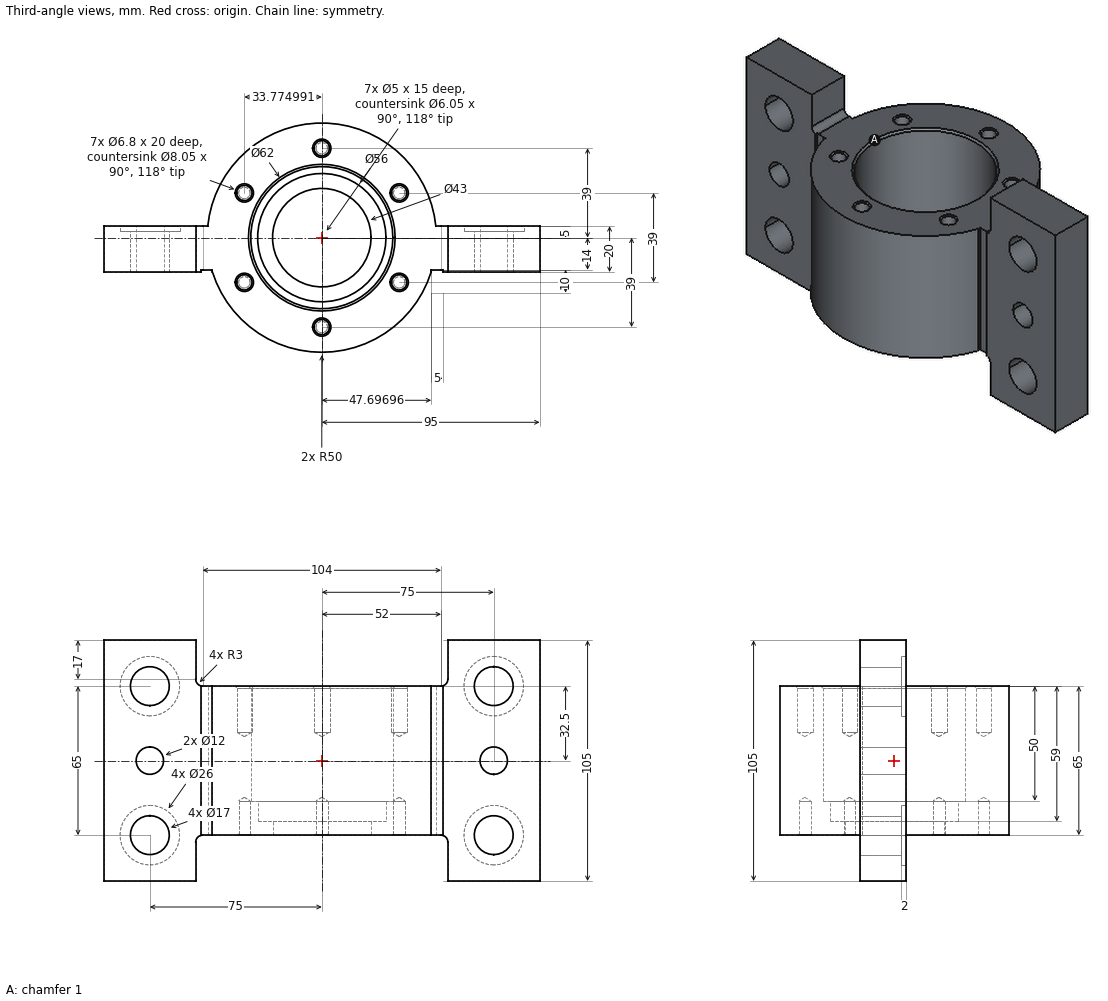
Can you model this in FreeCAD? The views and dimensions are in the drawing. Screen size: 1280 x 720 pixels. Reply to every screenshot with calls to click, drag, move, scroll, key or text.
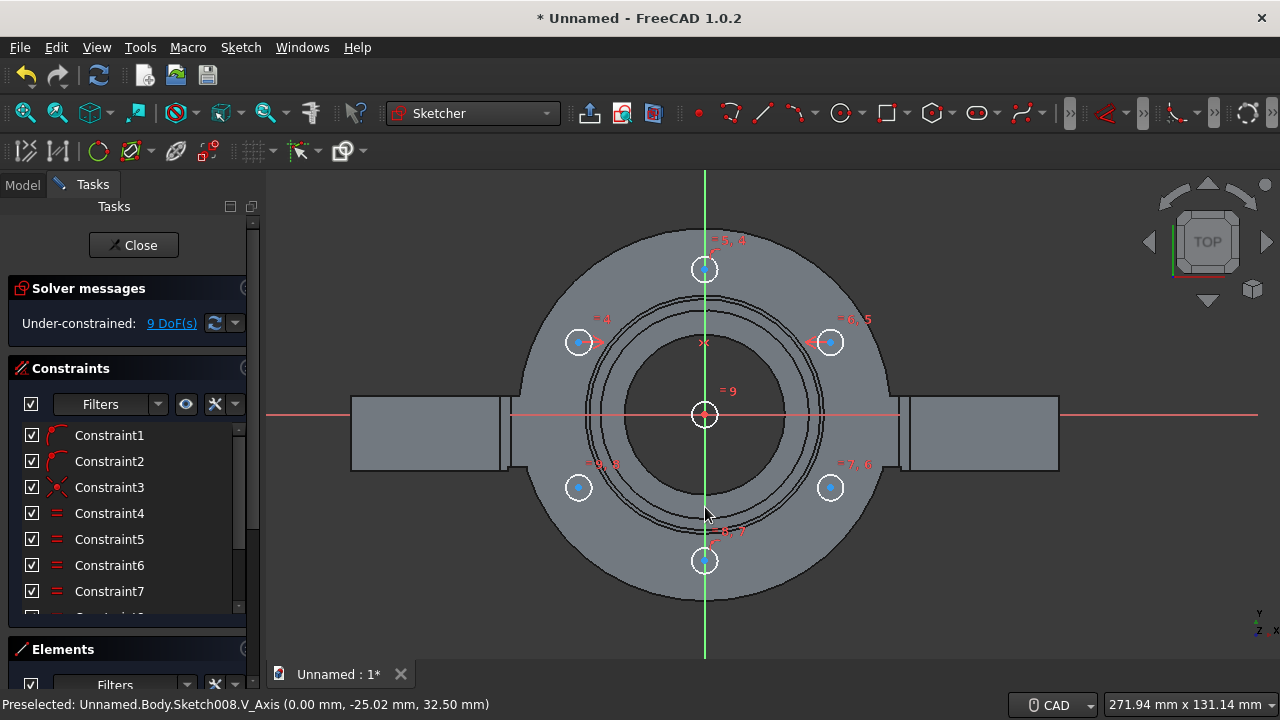
click(831, 342)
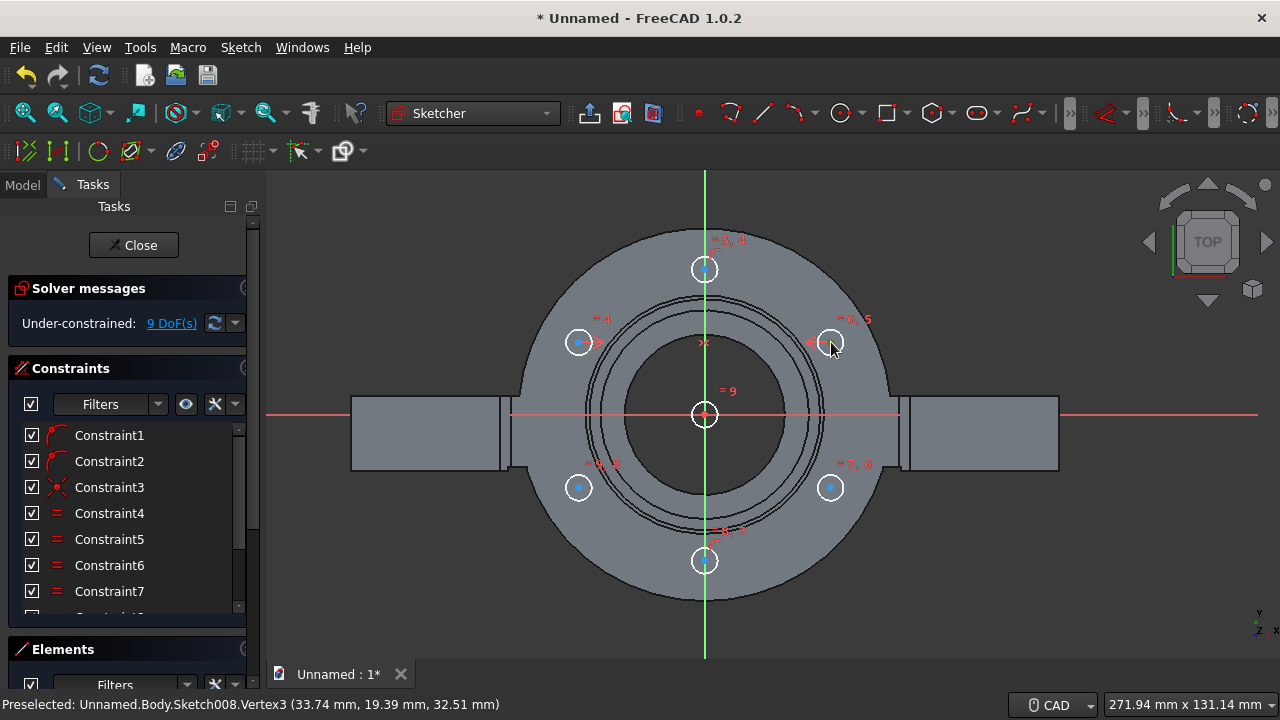
click(831, 488)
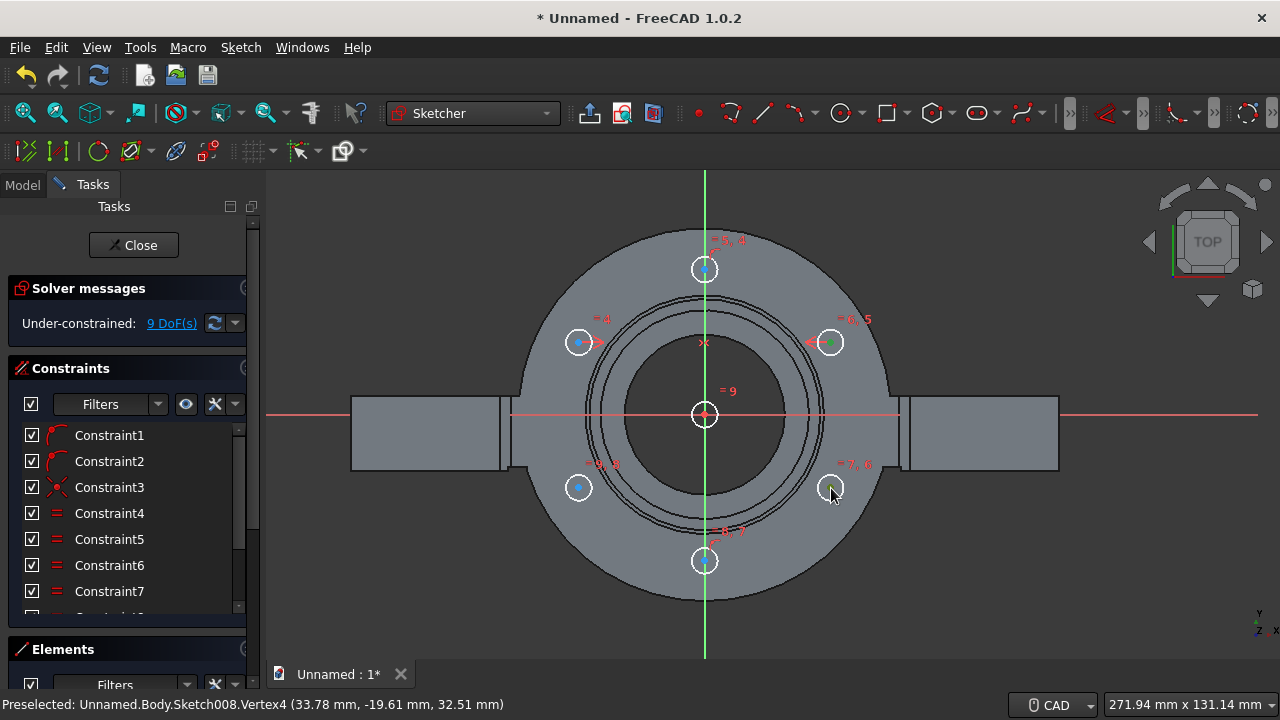
click(353, 415)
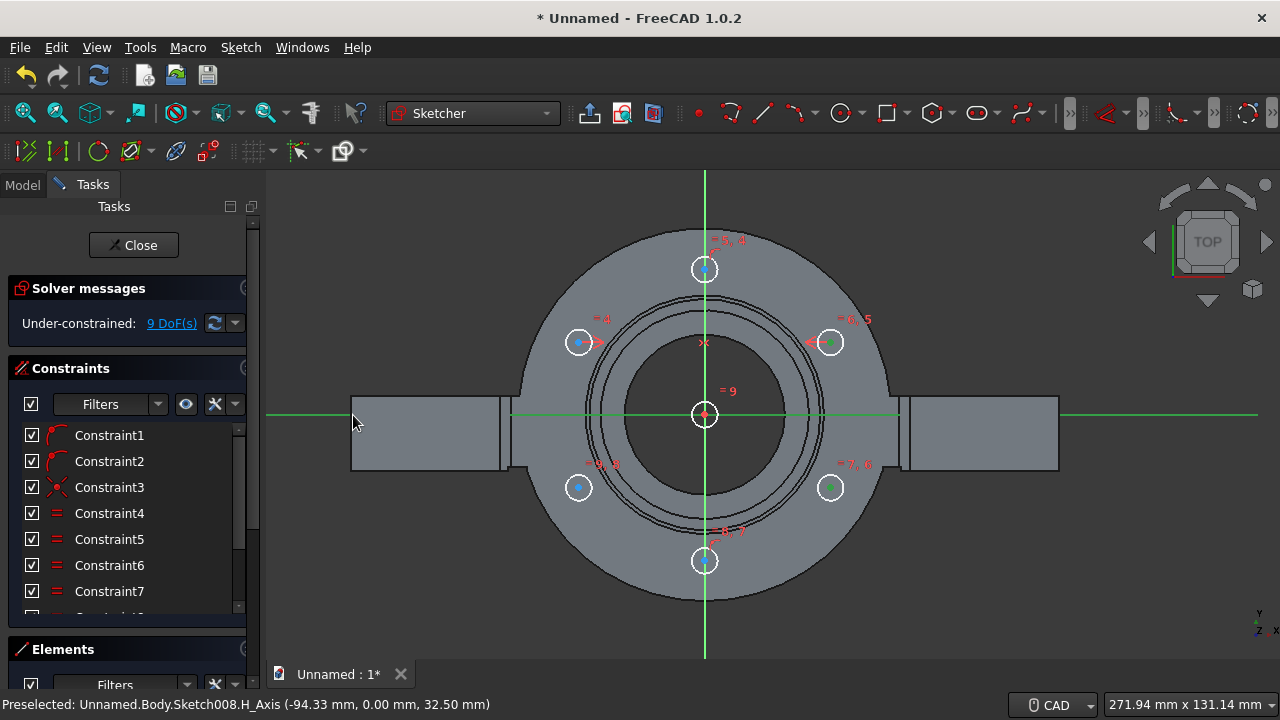
key(s)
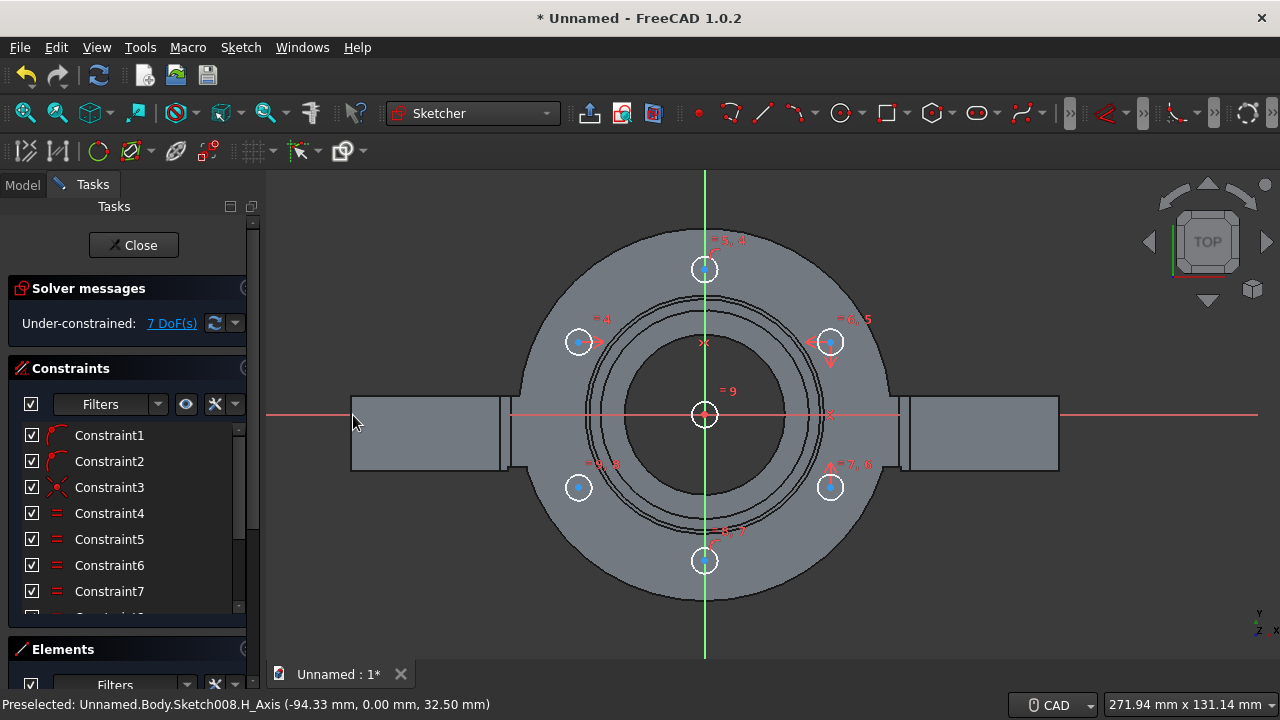
click(579, 342)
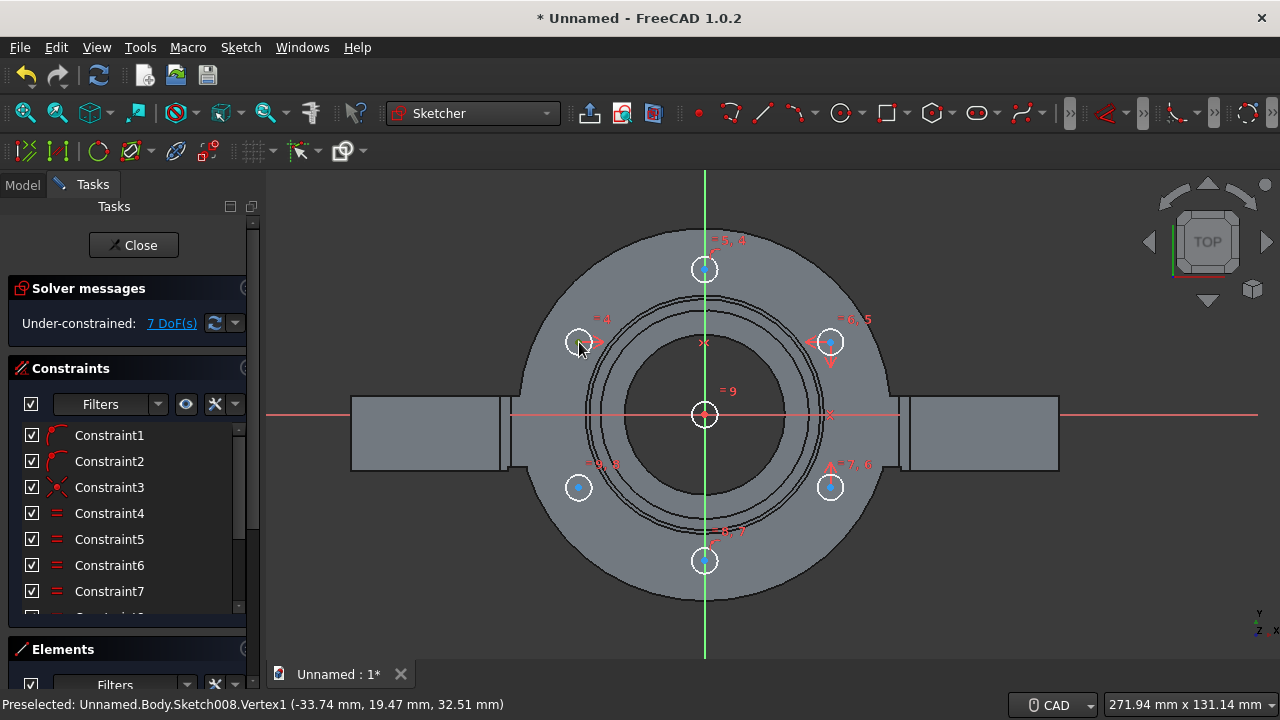
click(579, 488)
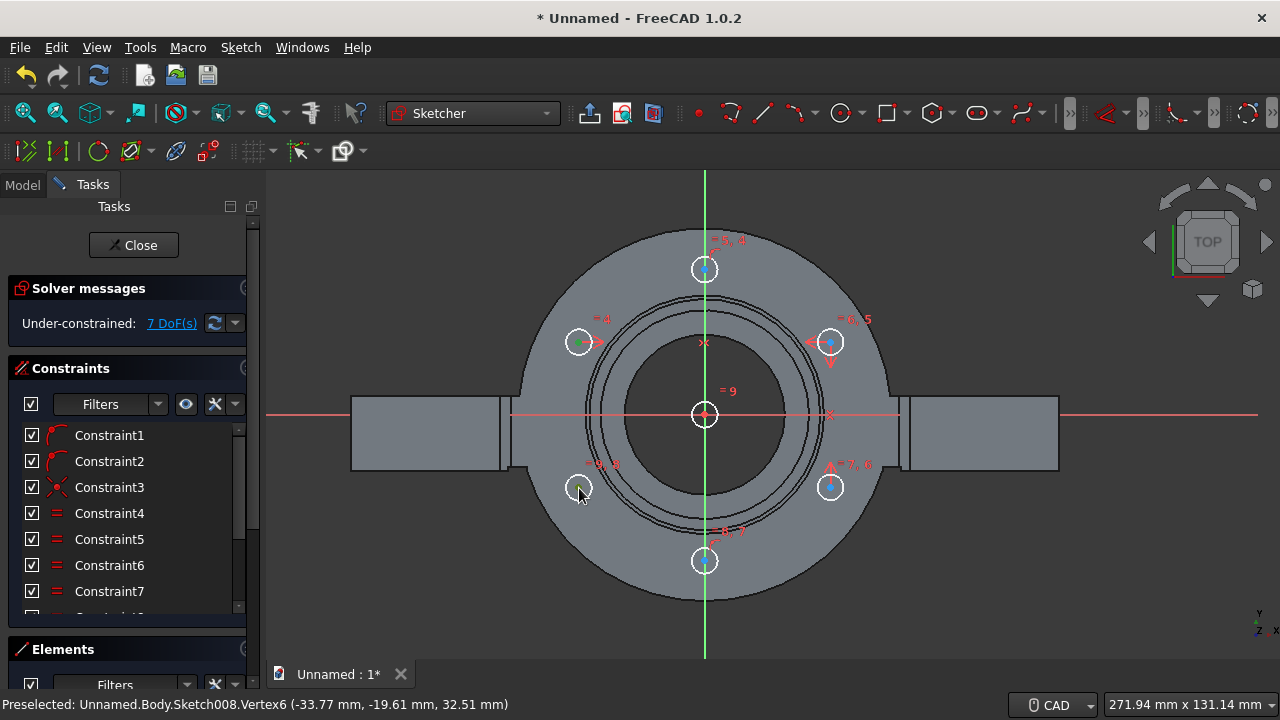
click(353, 415)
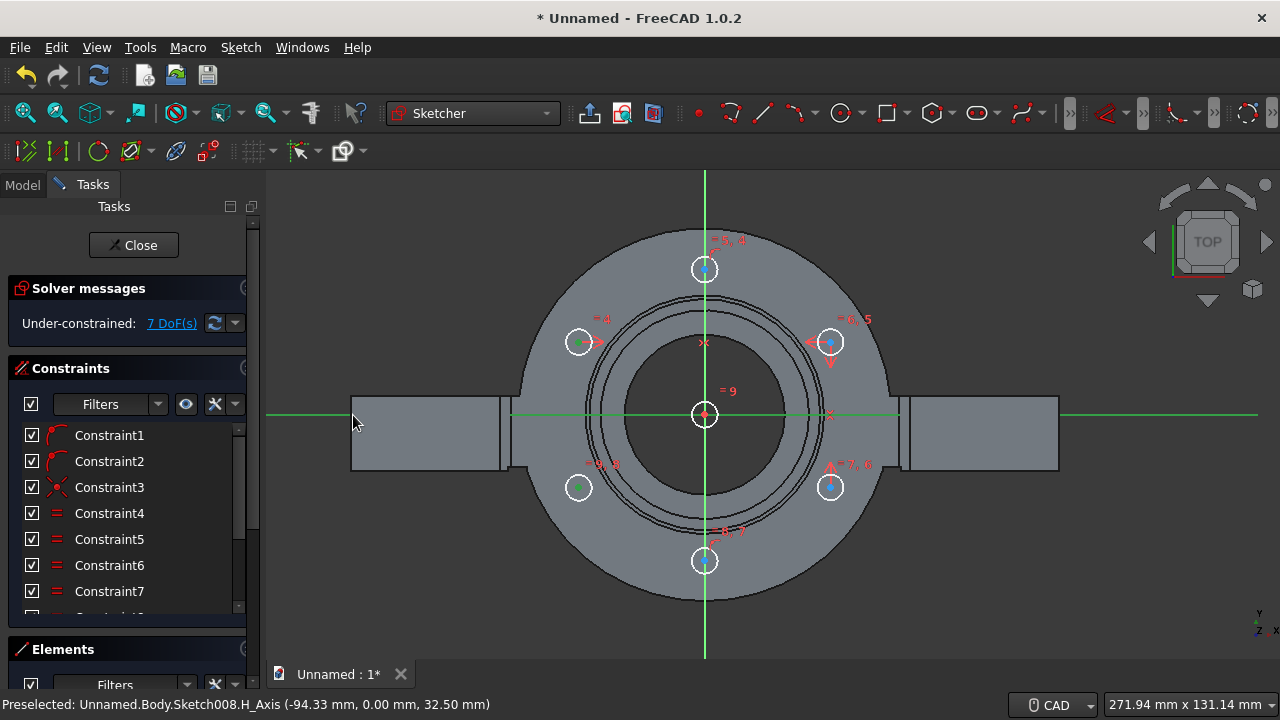
key(s)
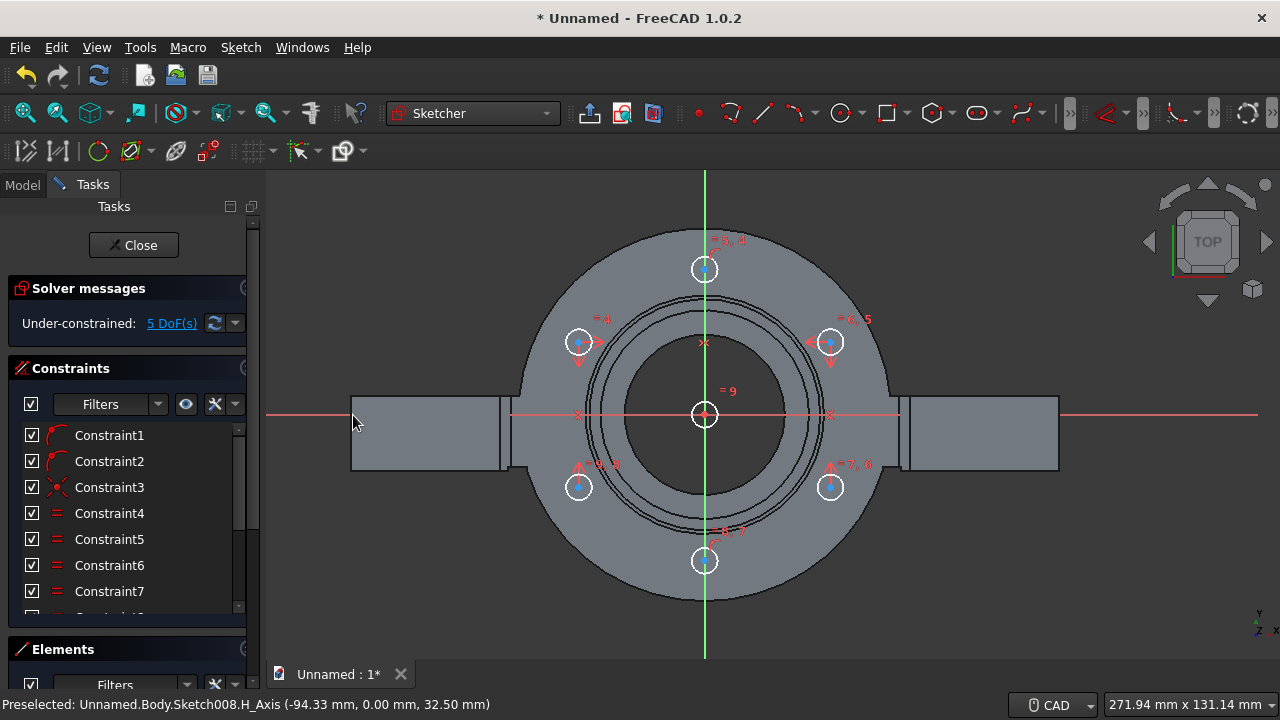
click(1106, 114)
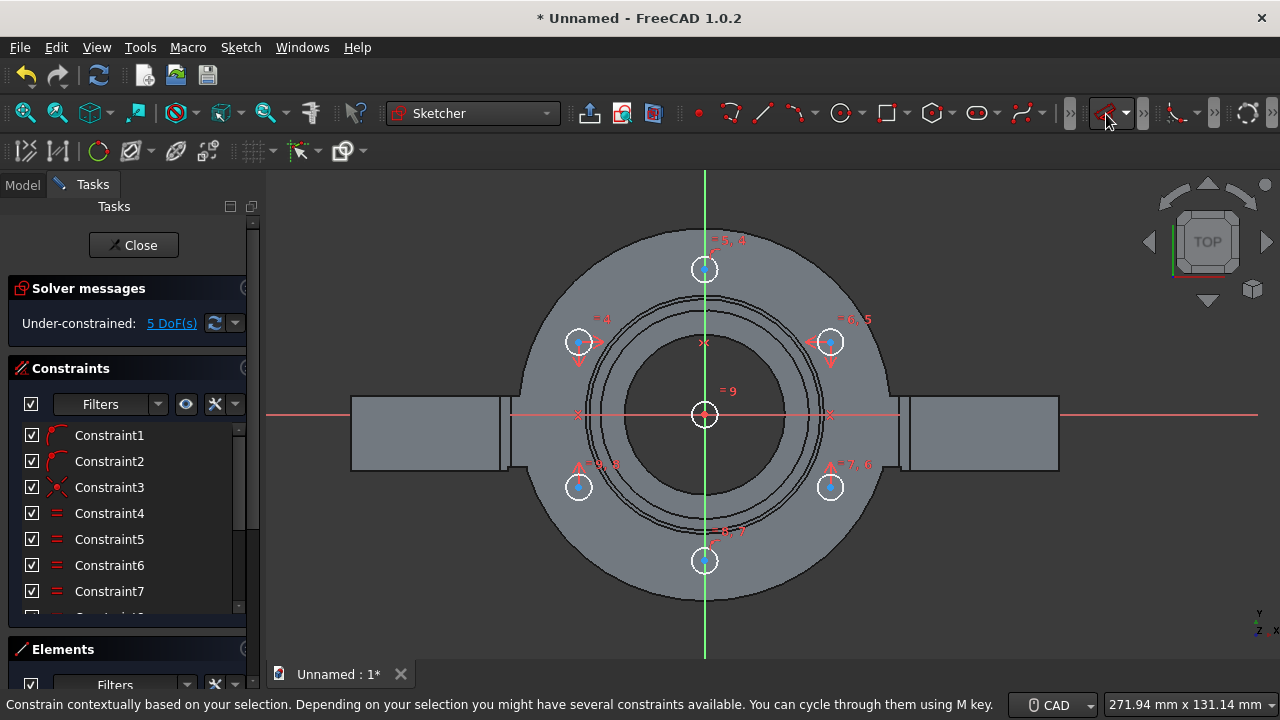
scroll(588, 333, up, 3)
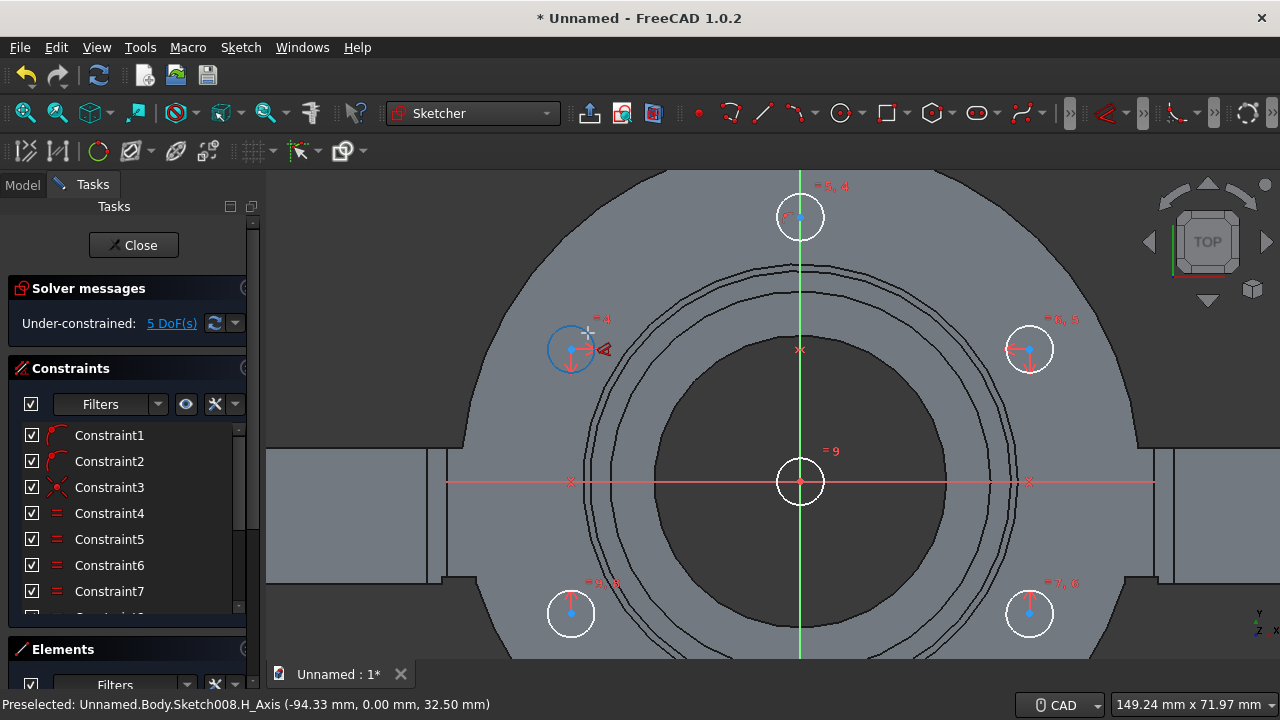
click(588, 333)
click(611, 311)